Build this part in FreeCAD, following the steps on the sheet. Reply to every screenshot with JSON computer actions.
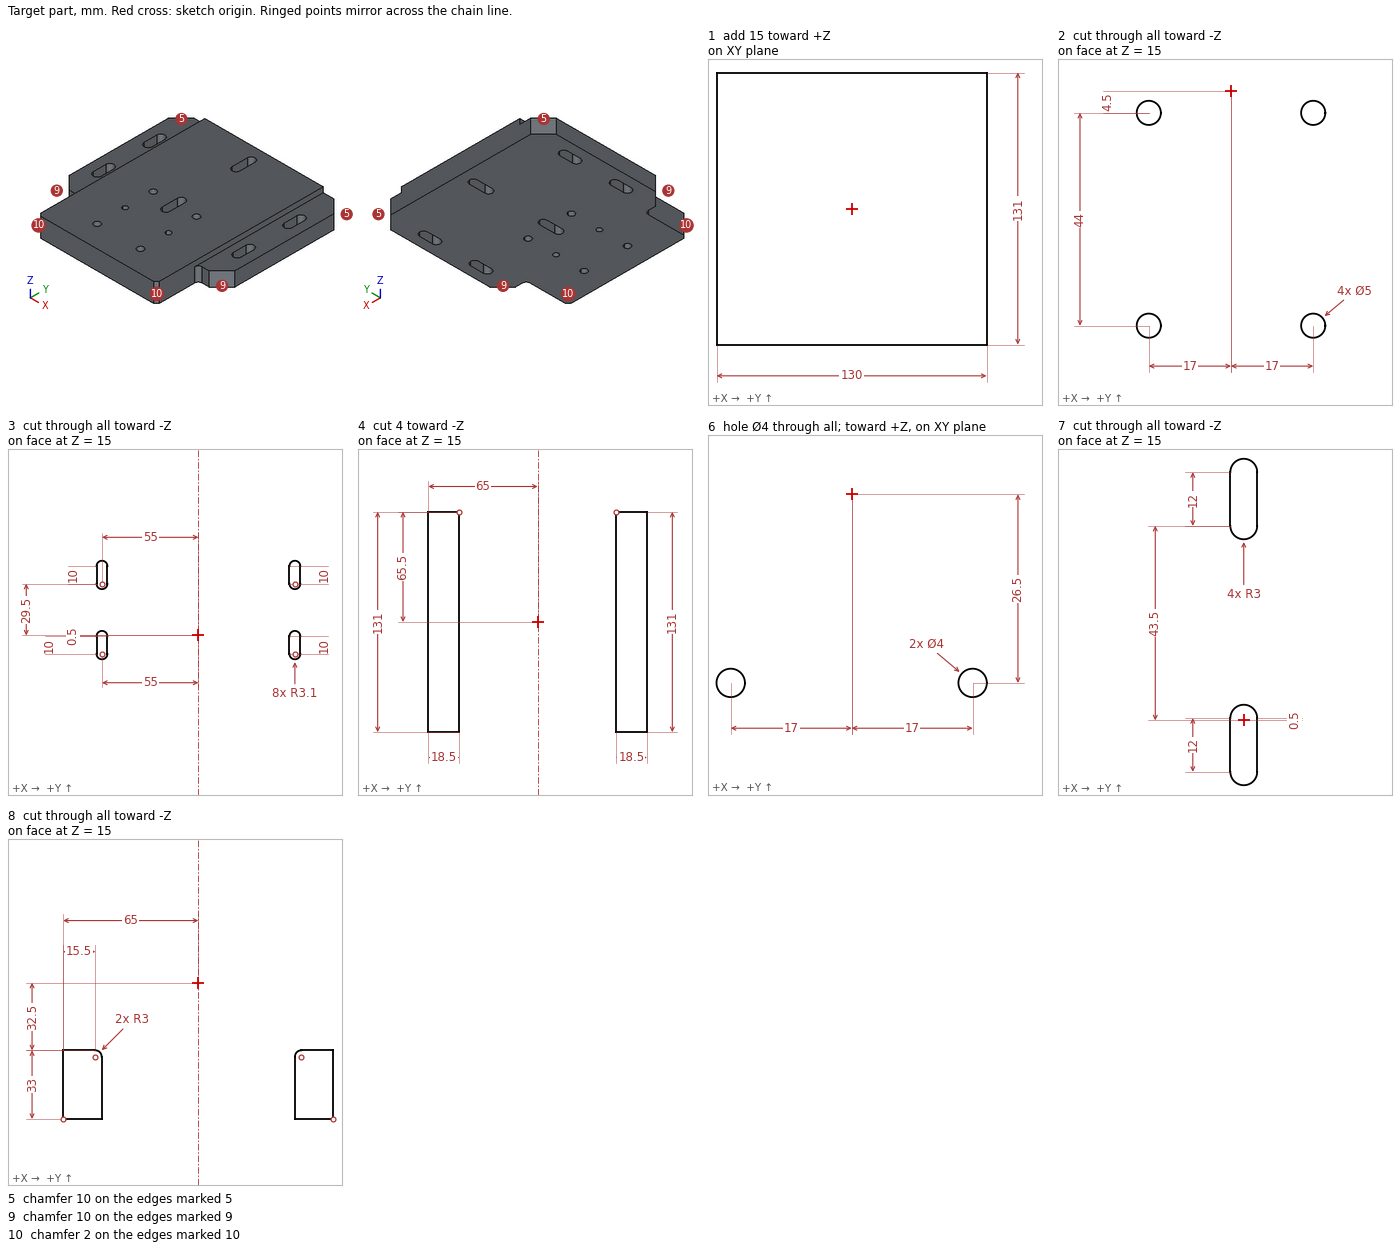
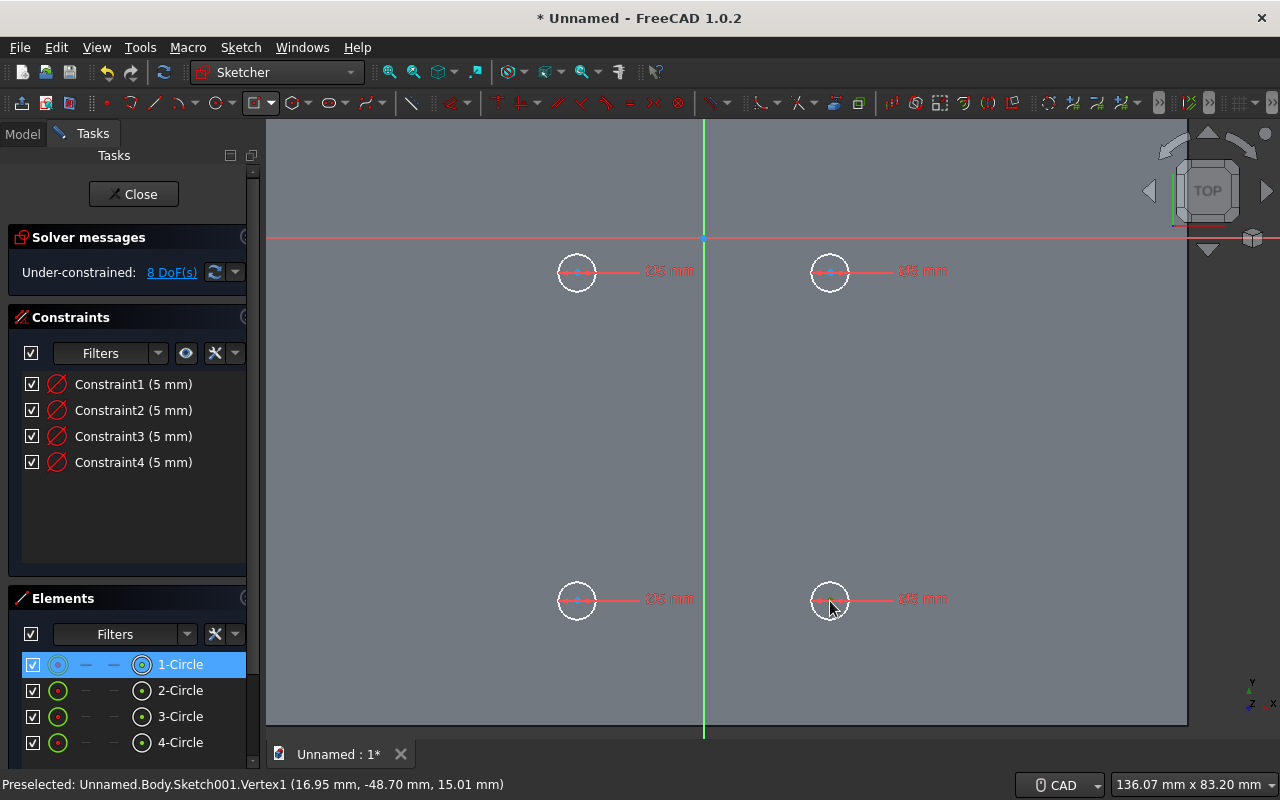
{"action": "left_click", "coordinate": [577, 601]}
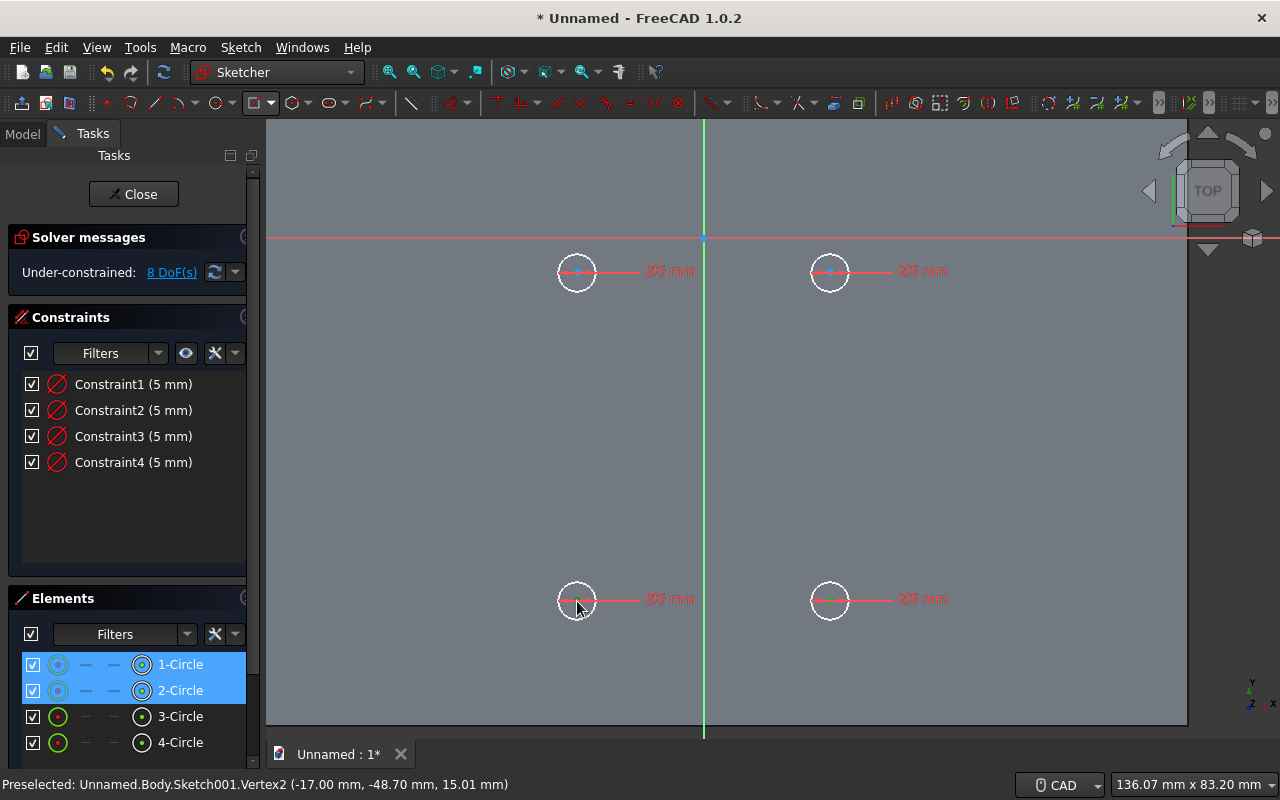
{"action": "key", "text": "h"}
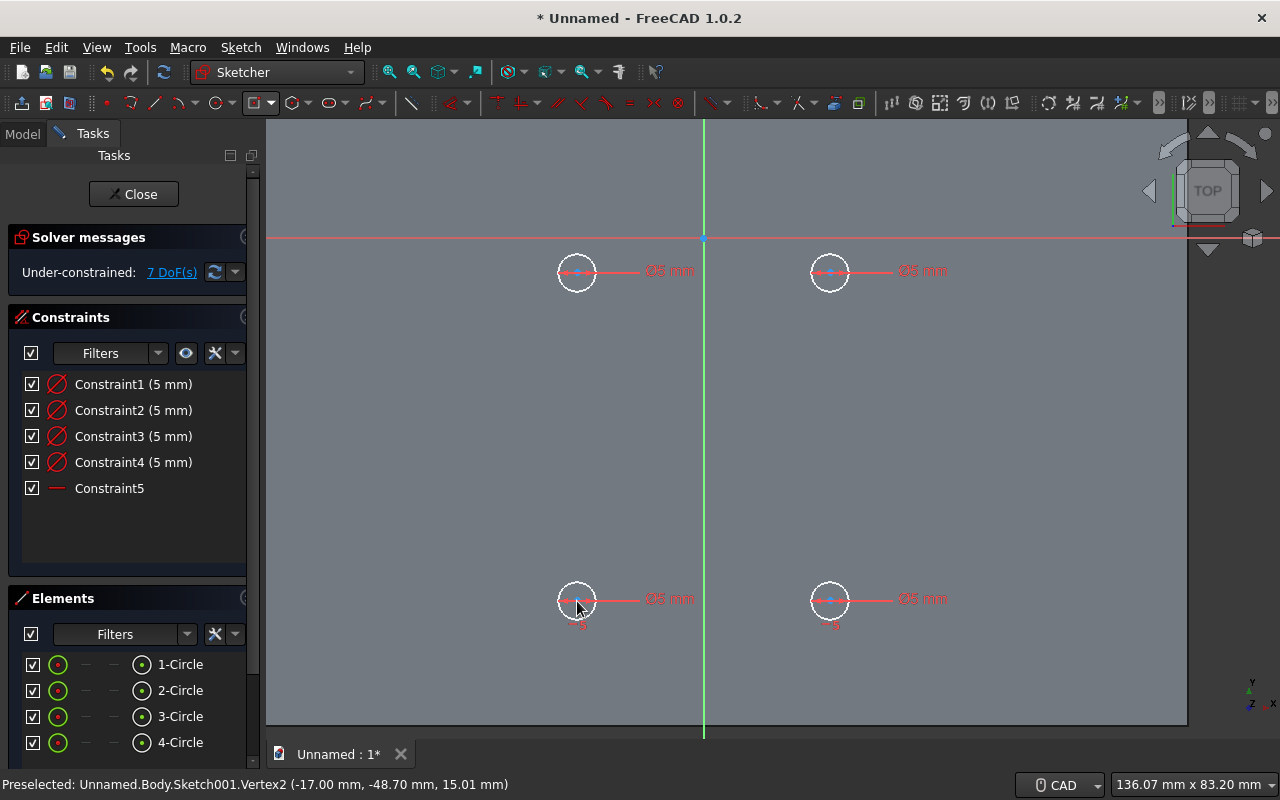
{"action": "left_click", "coordinate": [577, 601]}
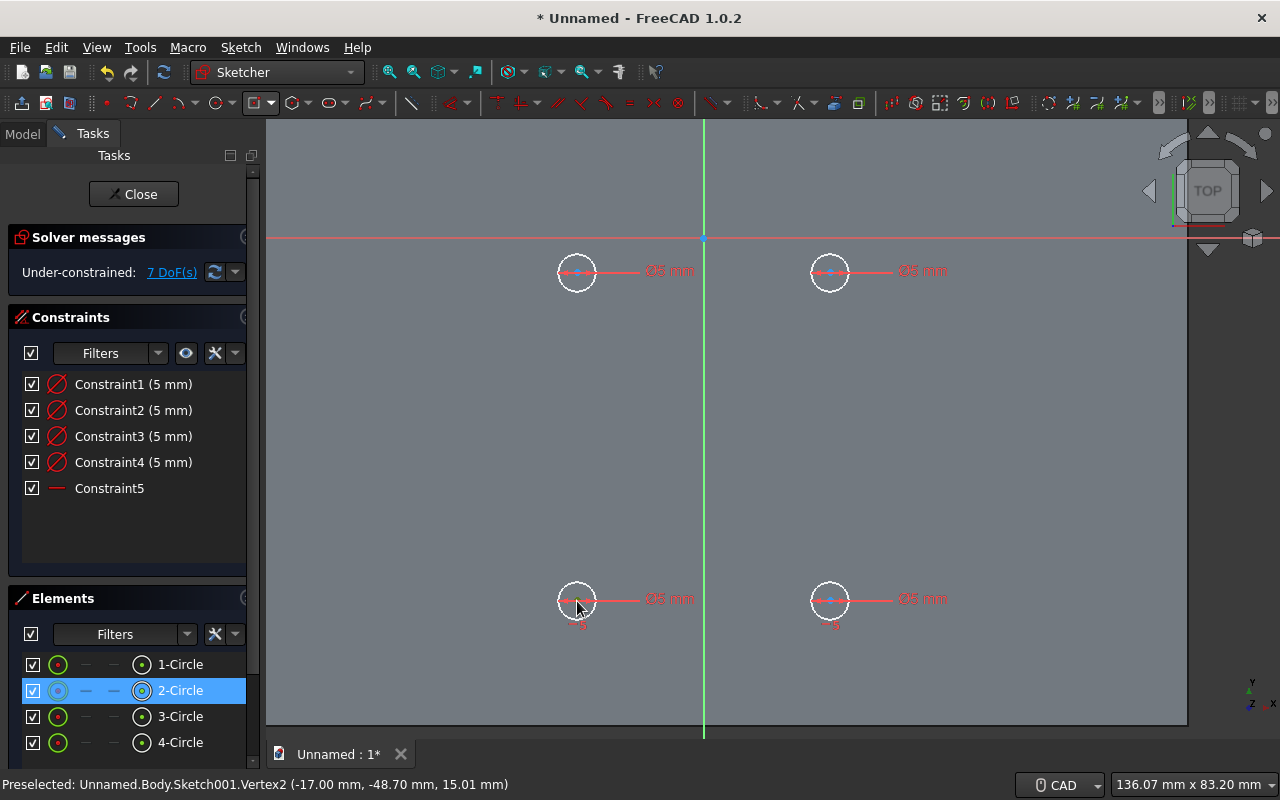
{"action": "left_click", "coordinate": [577, 273]}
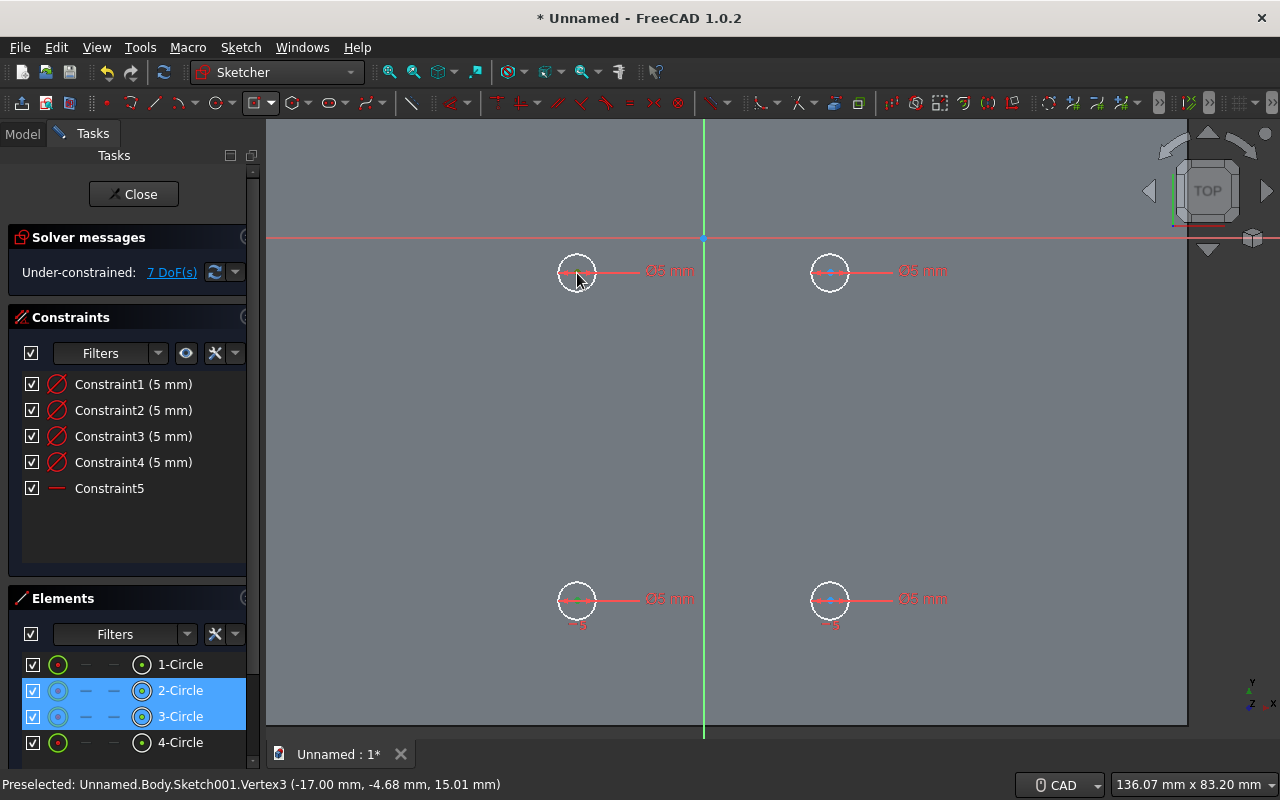
{"action": "key", "text": "v"}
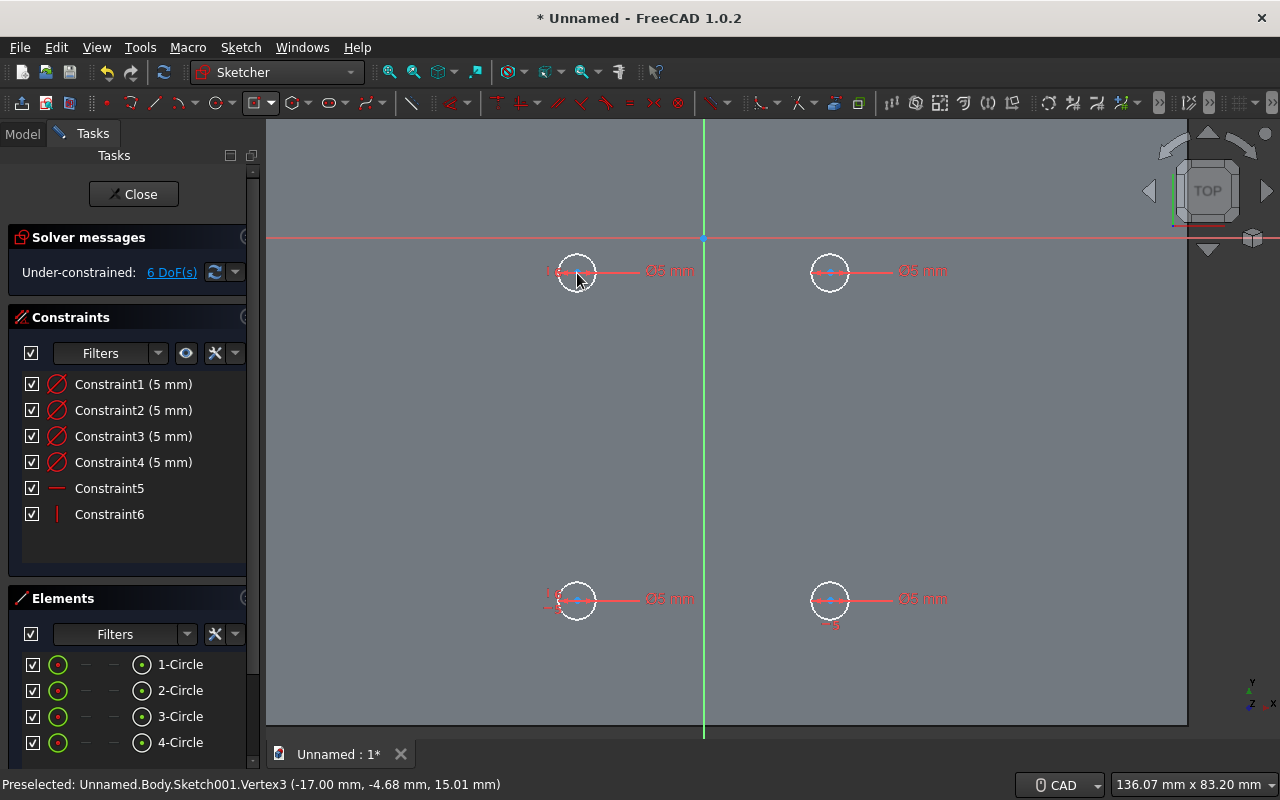
{"action": "left_click", "coordinate": [830, 601]}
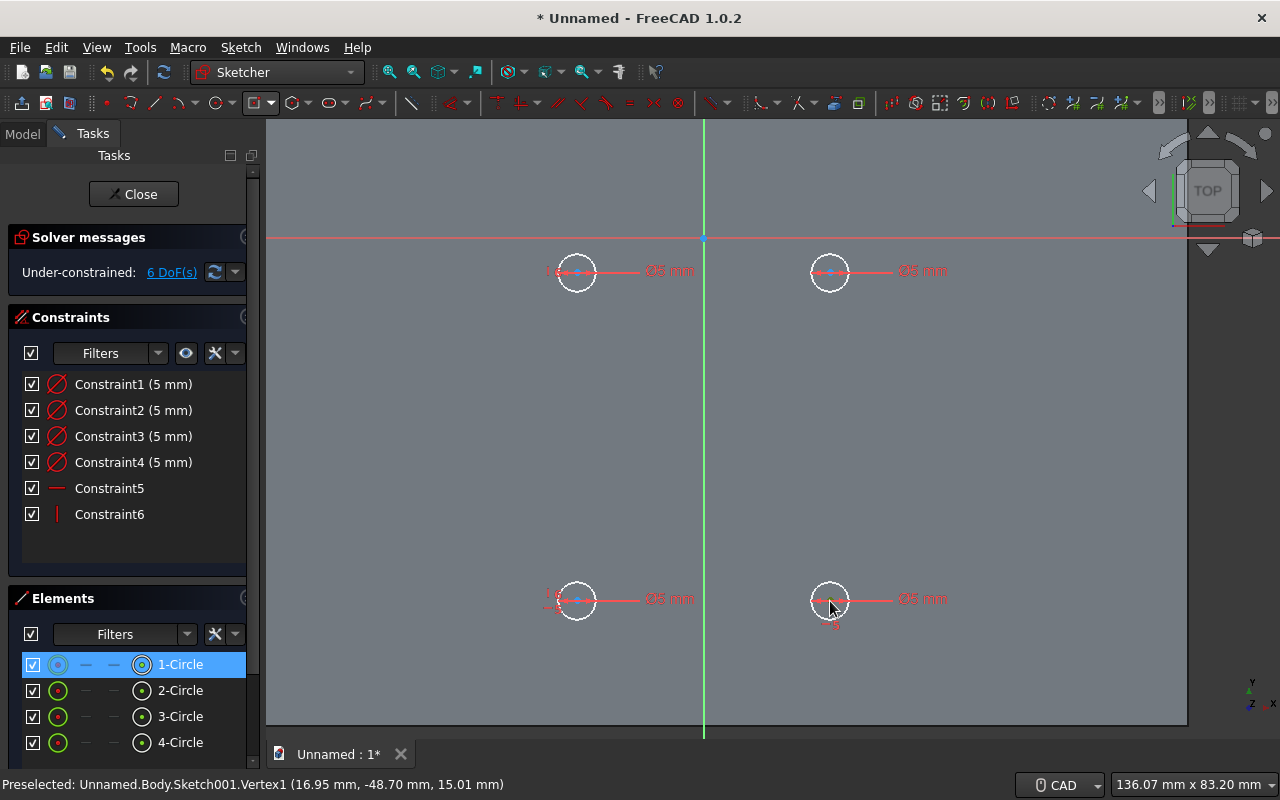
{"action": "left_click", "coordinate": [830, 273]}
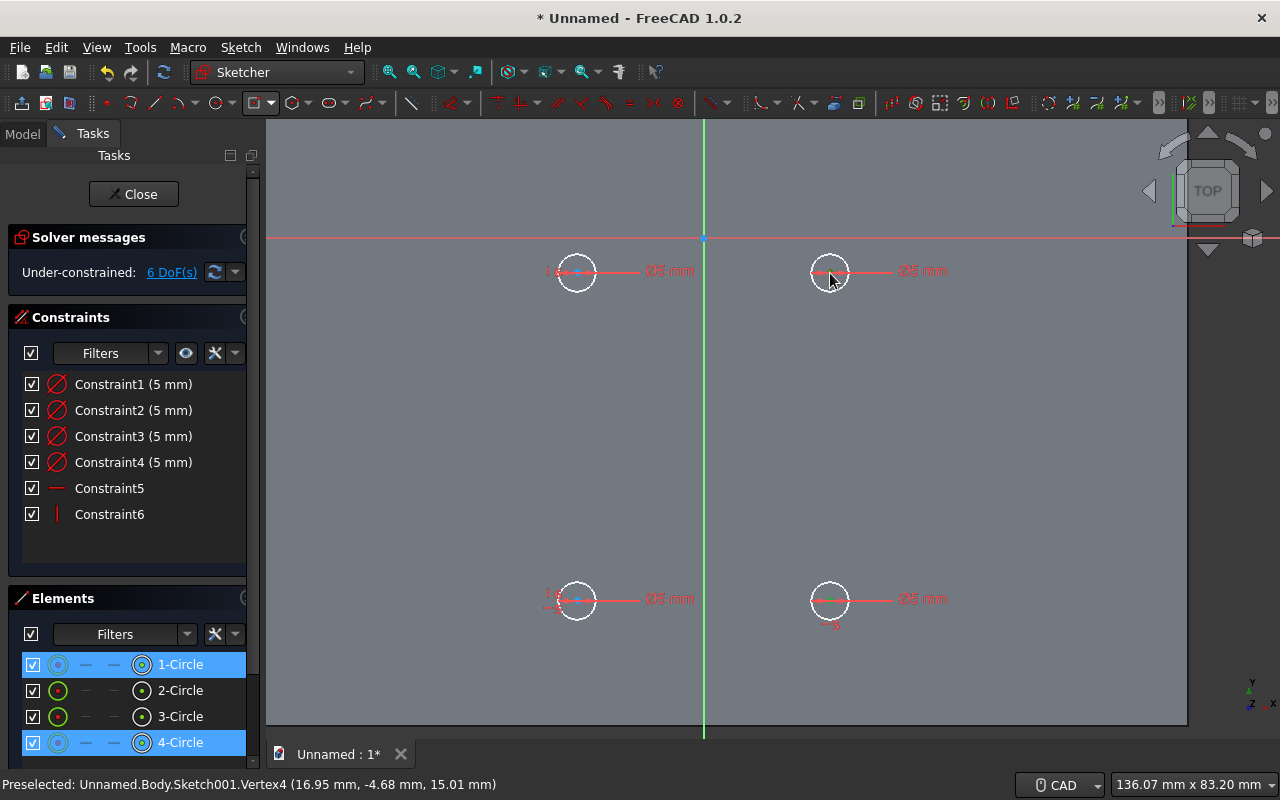
{"action": "key", "text": "v"}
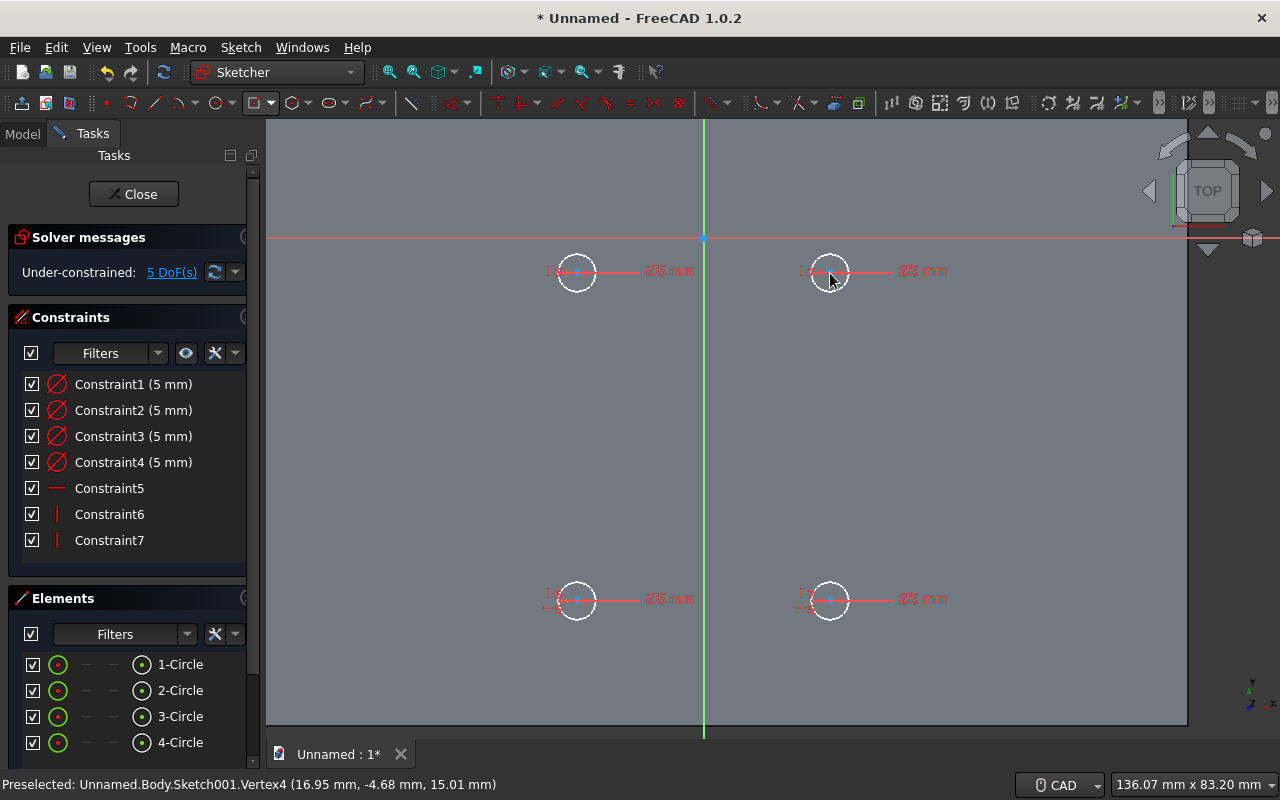
{"action": "left_click", "coordinate": [577, 273]}